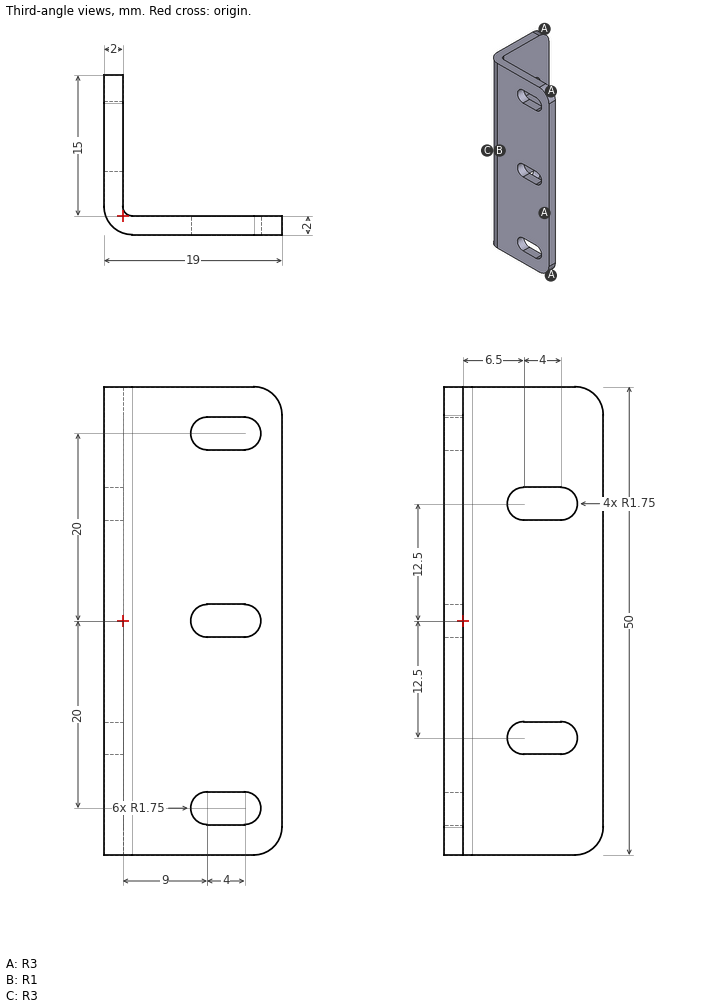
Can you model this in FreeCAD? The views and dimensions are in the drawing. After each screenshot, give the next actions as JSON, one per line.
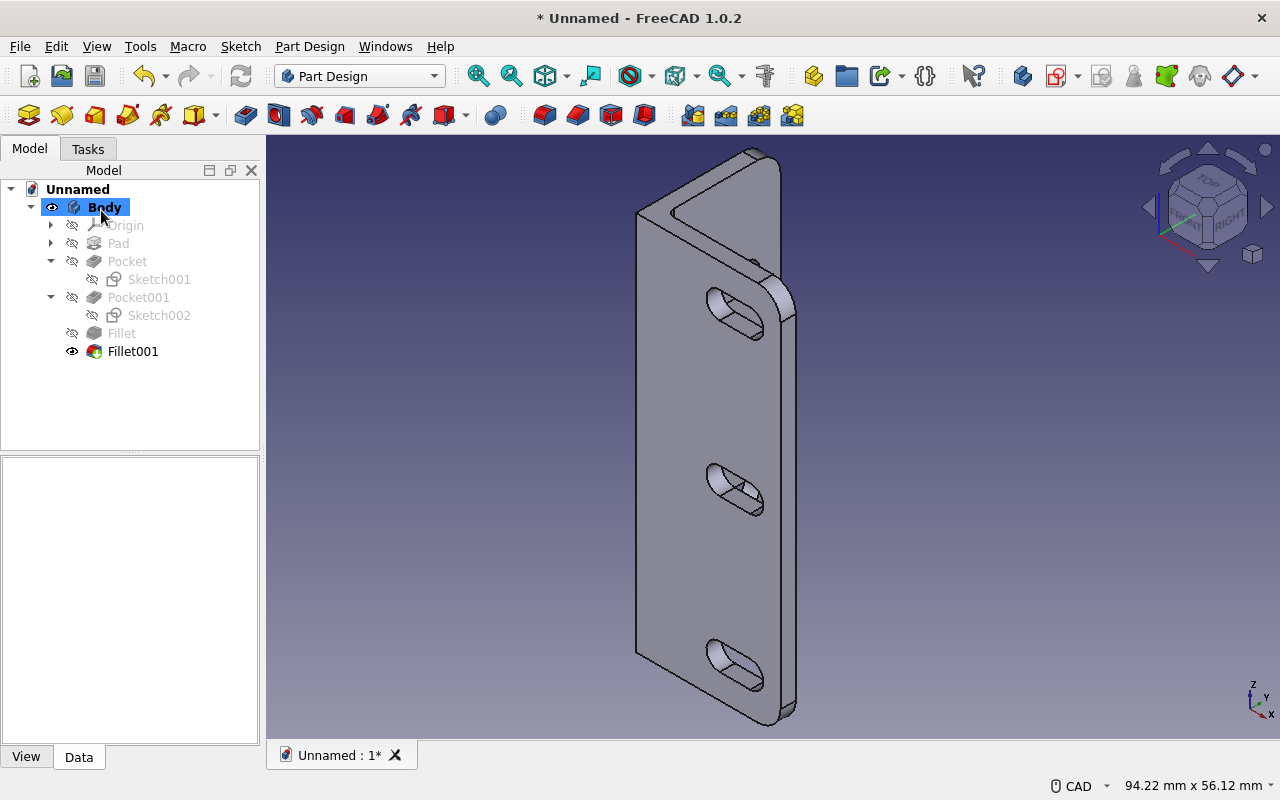
{"action": "key", "text": "2"}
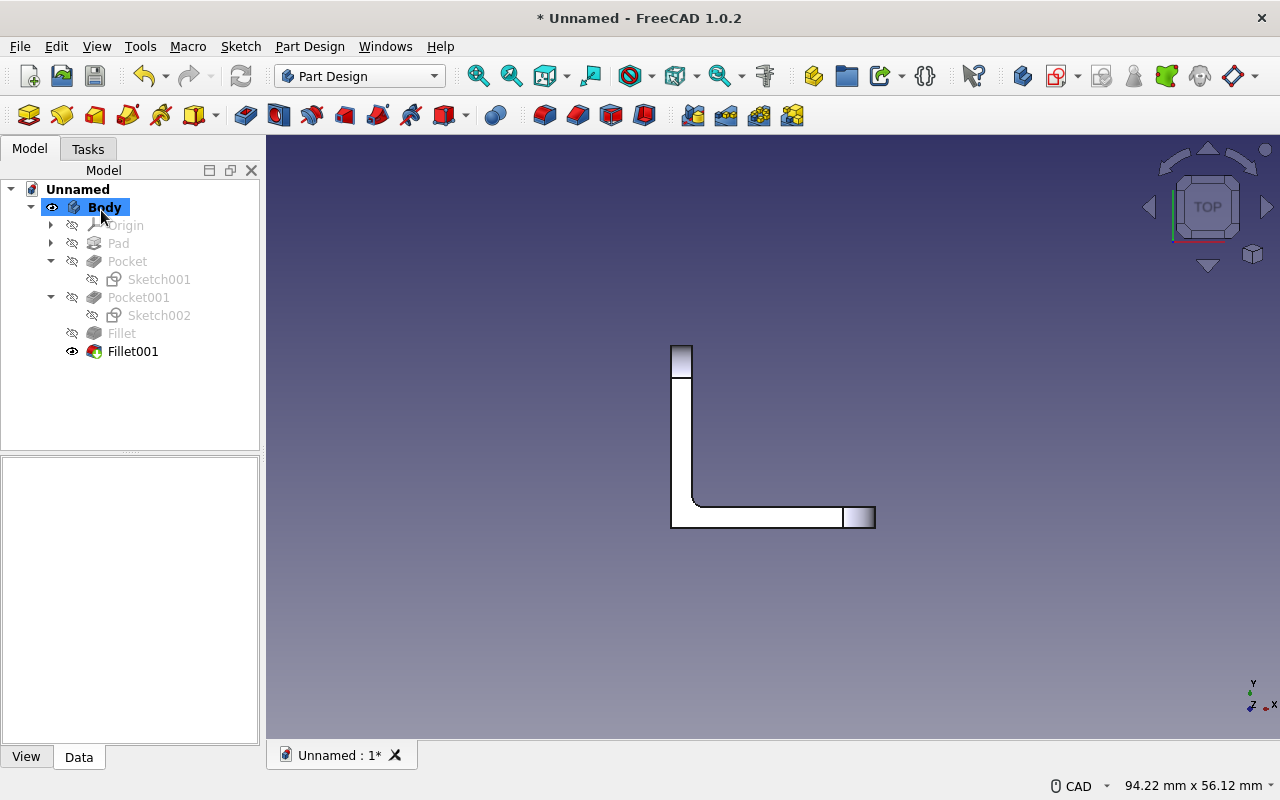
{"action": "left_click", "coordinate": [479, 76]}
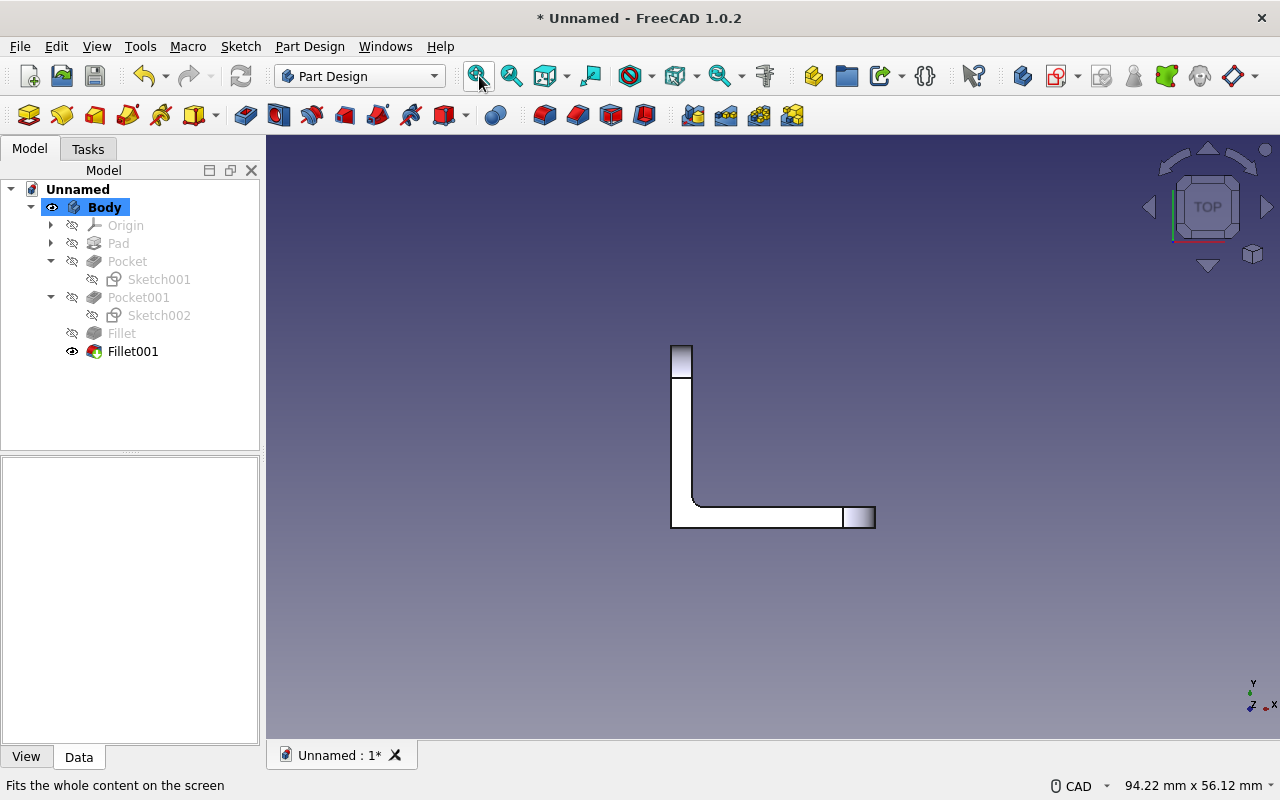
{"action": "key", "text": "0"}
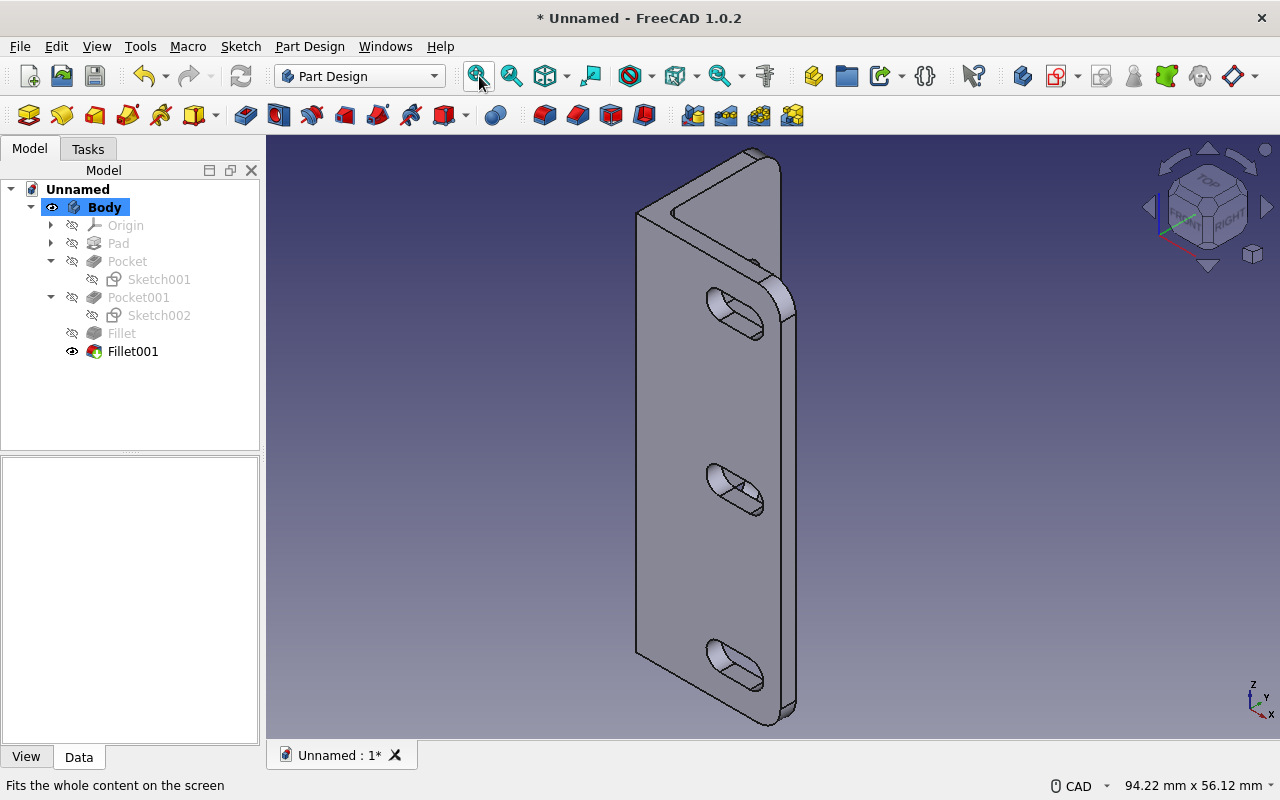
{"action": "key", "text": "1"}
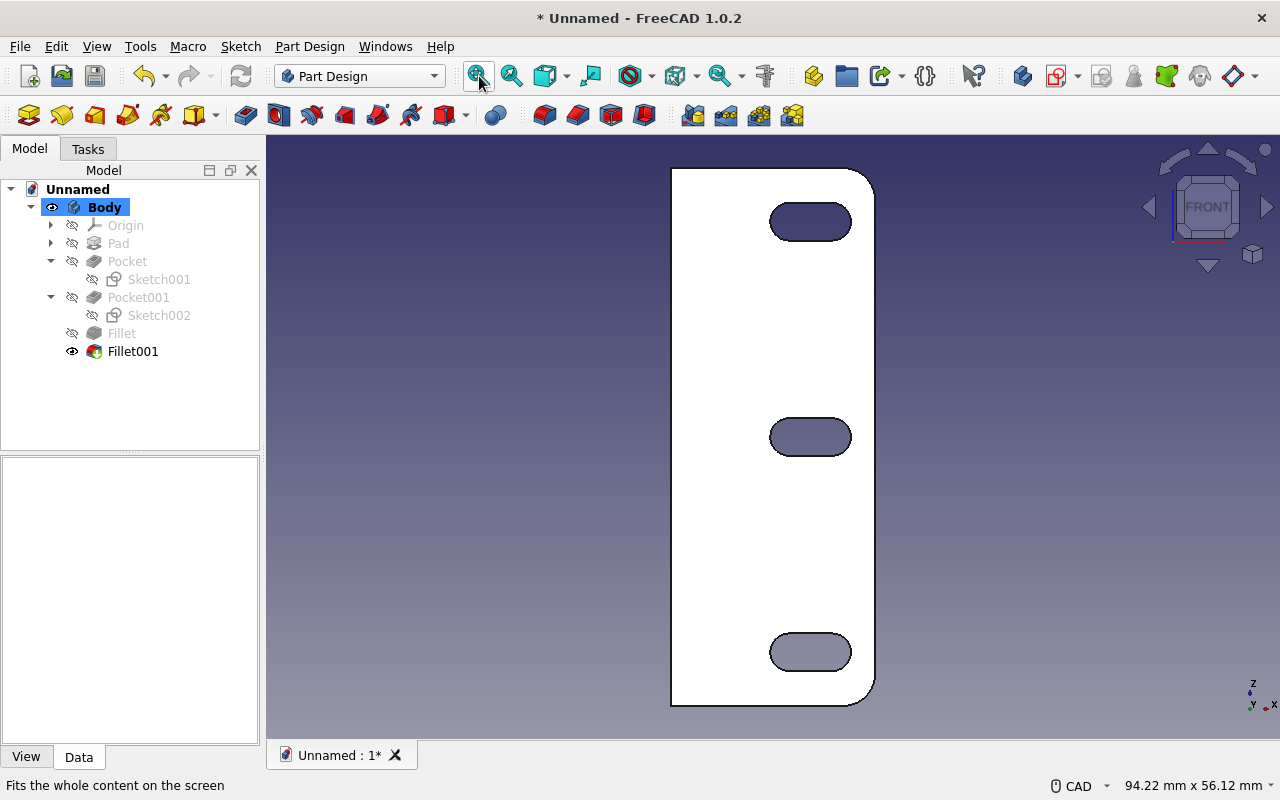
{"action": "left_click", "coordinate": [671, 436]}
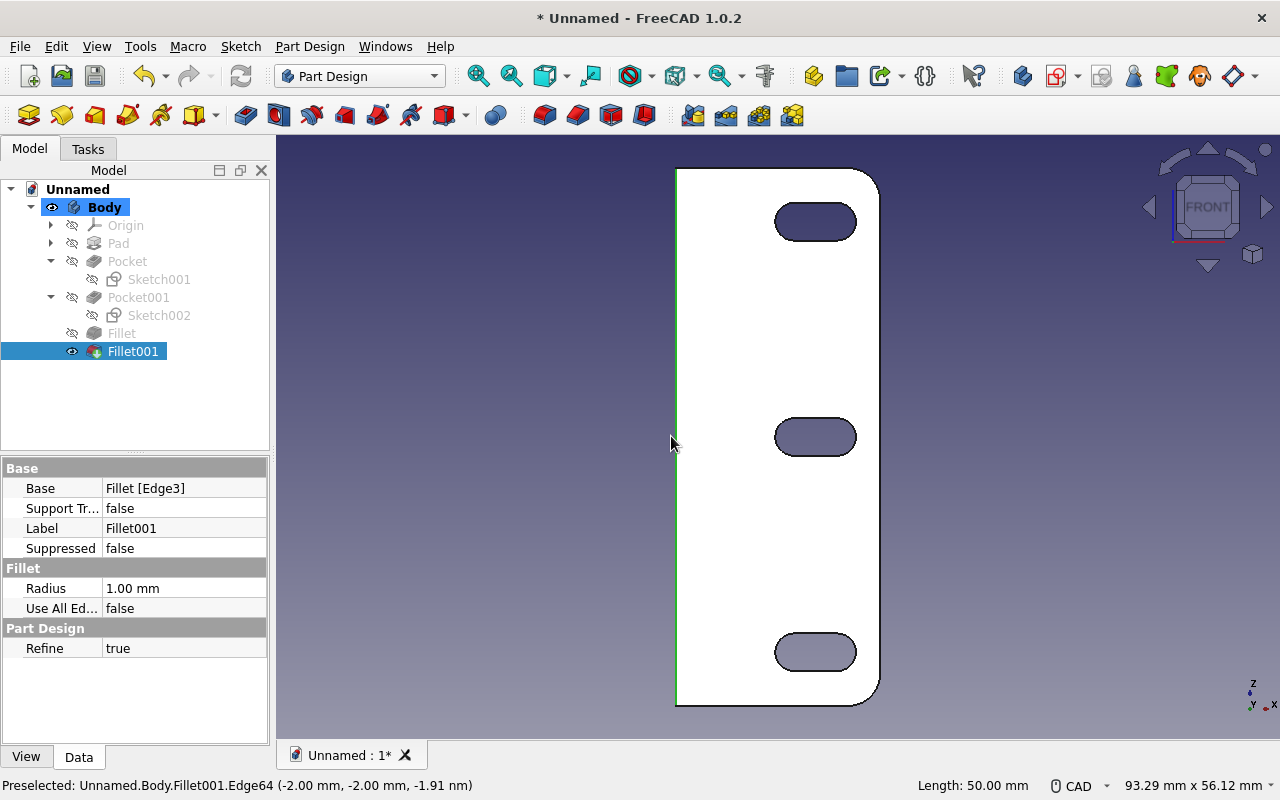
{"action": "left_click", "coordinate": [545, 116]}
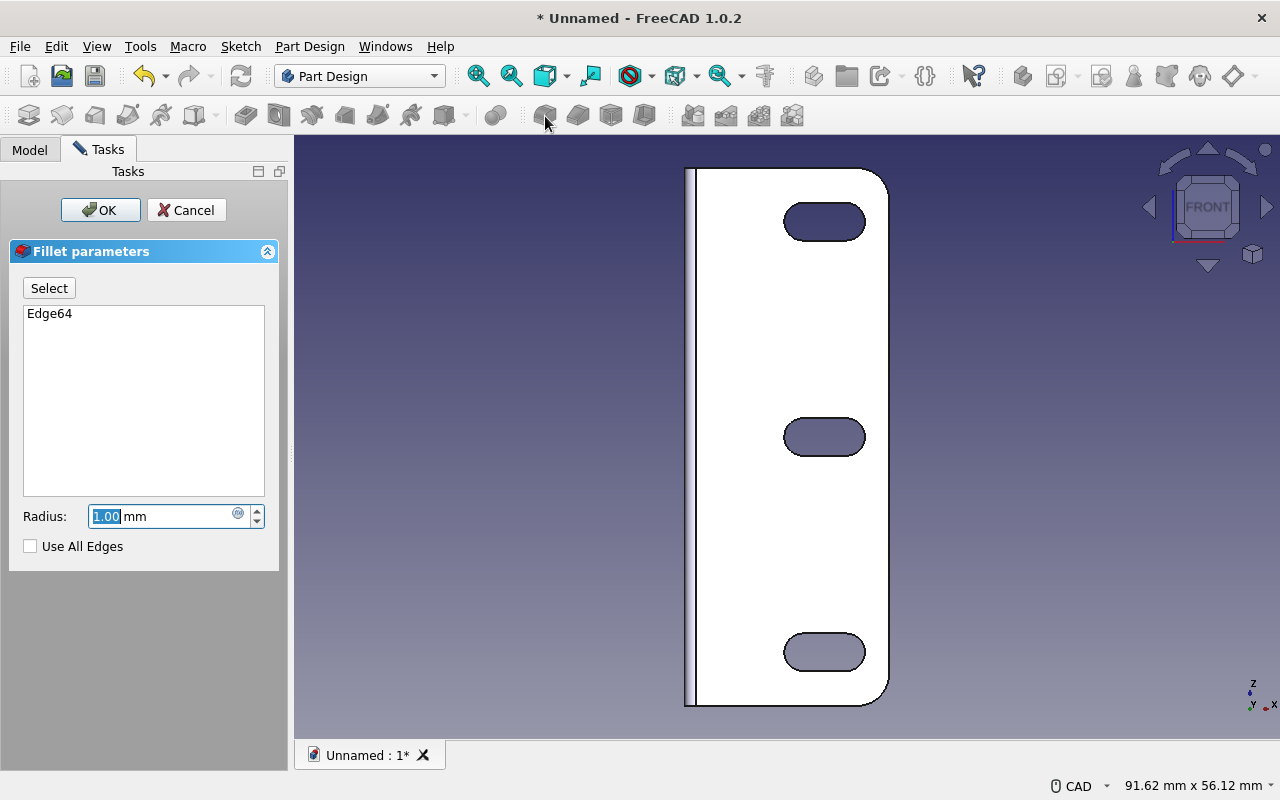
{"action": "type", "text": "3"}
{"action": "key", "text": "Tab"}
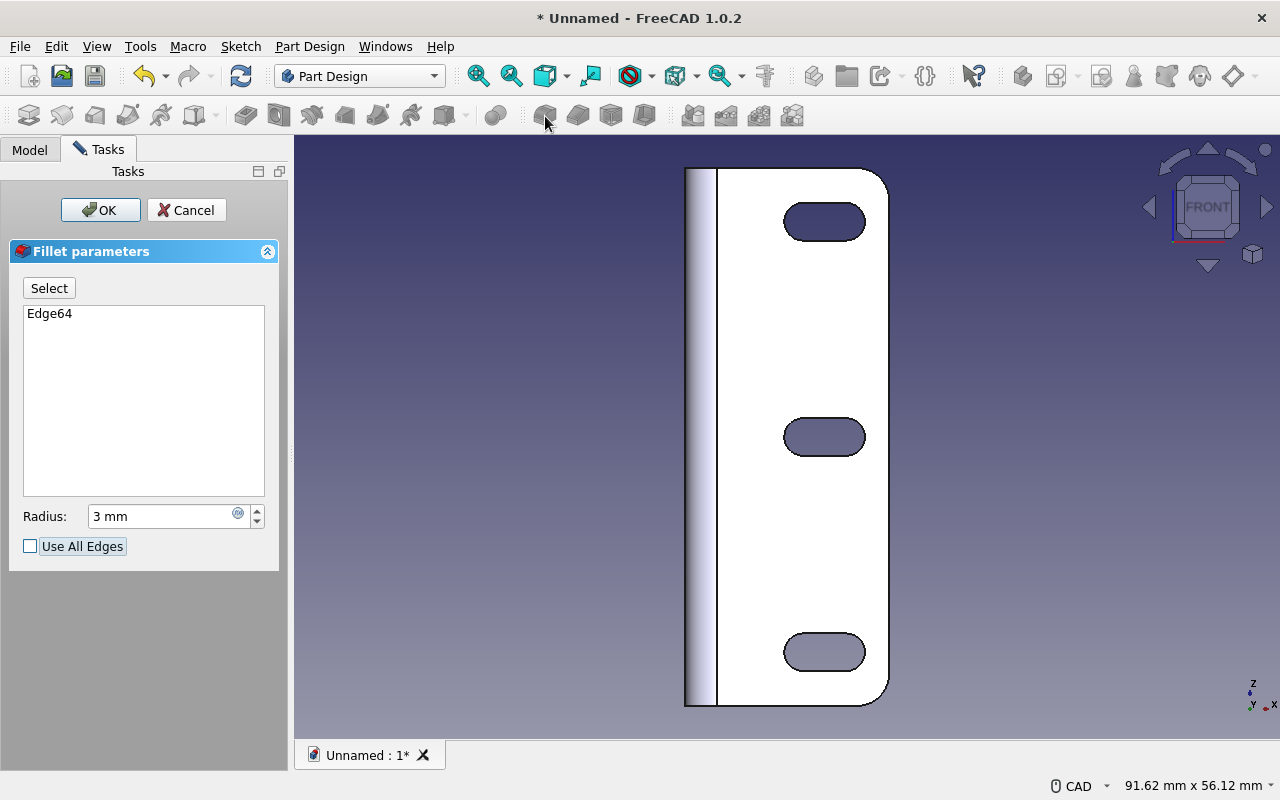
{"action": "left_click", "coordinate": [101, 210]}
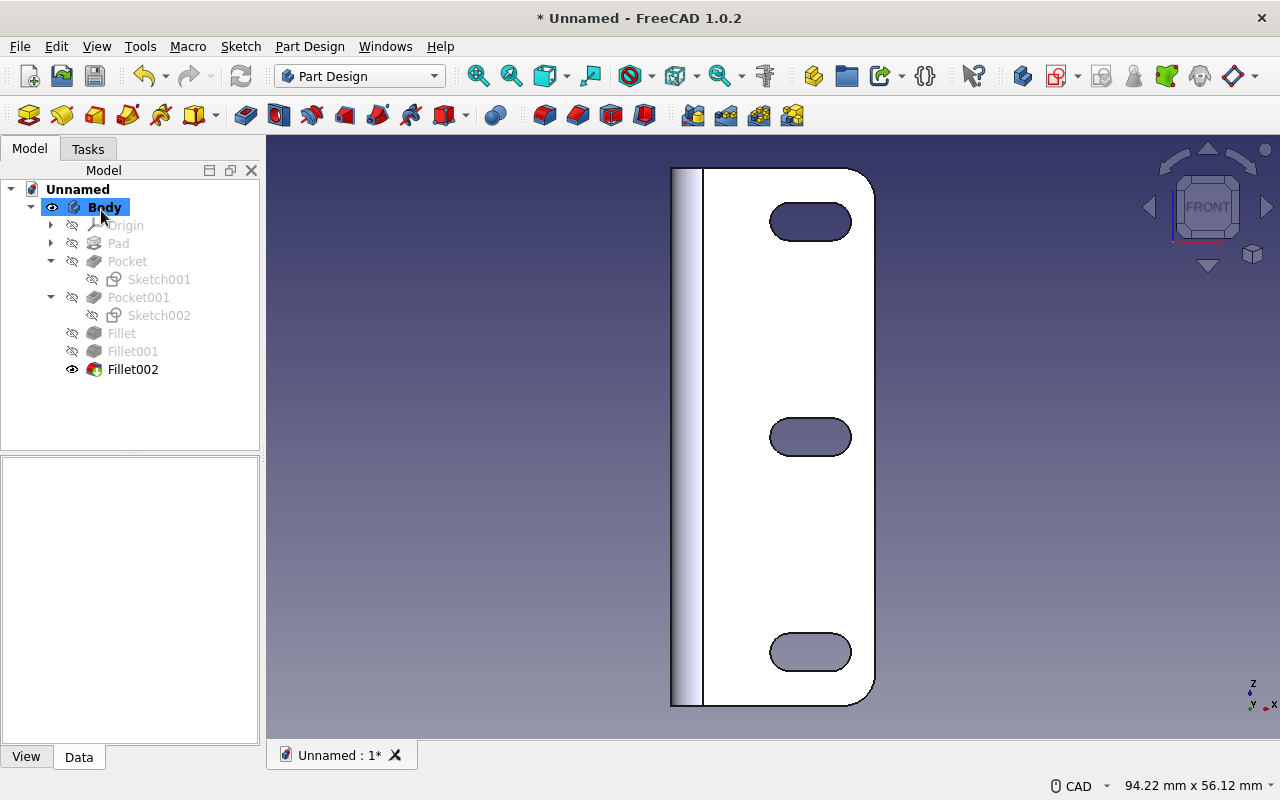
{"action": "key", "text": "0"}